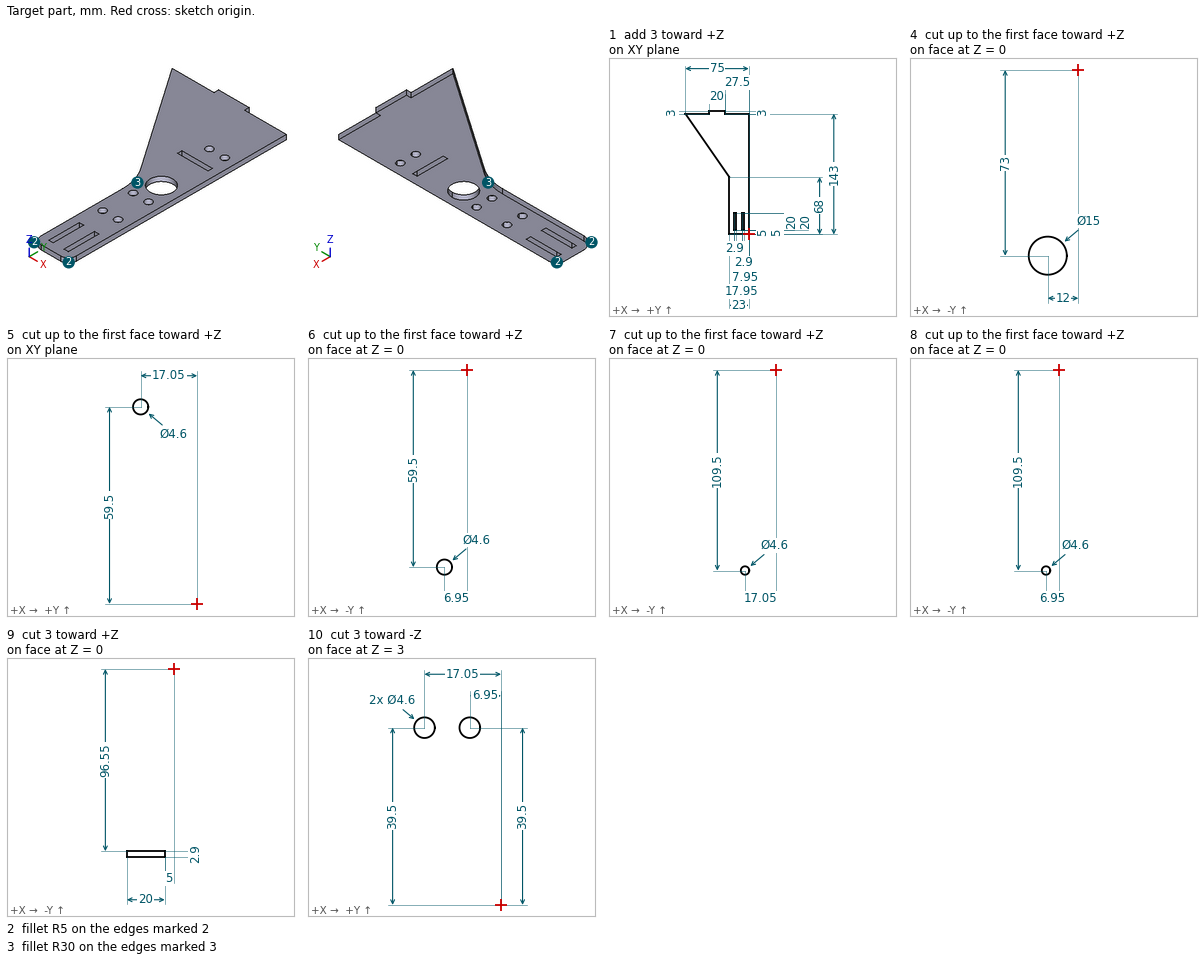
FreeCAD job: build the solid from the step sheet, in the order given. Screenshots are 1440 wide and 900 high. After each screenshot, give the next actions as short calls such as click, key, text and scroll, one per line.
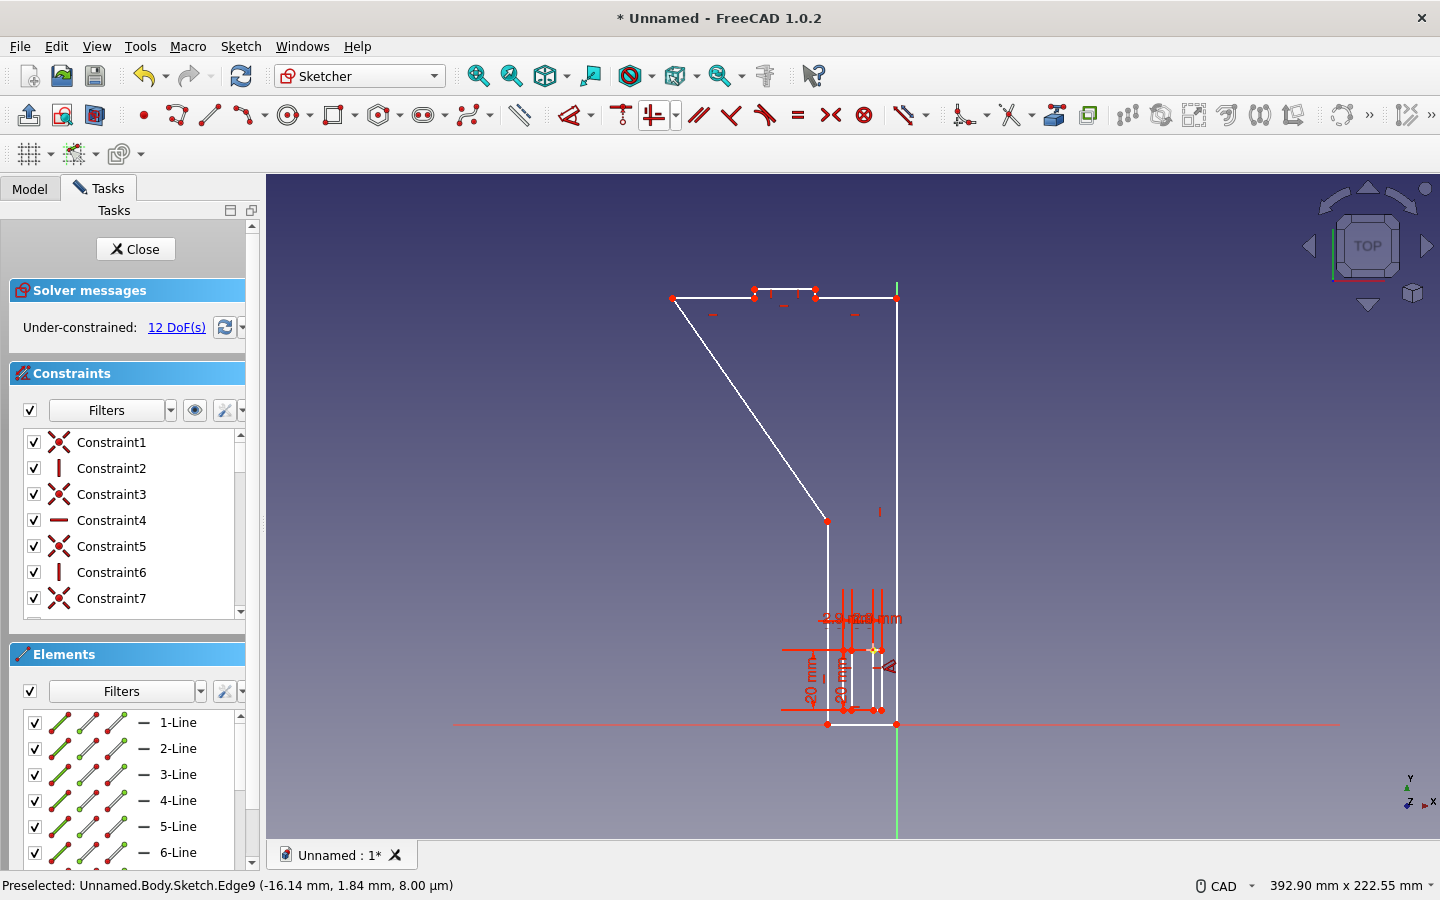
scroll(815, 294, up, 8)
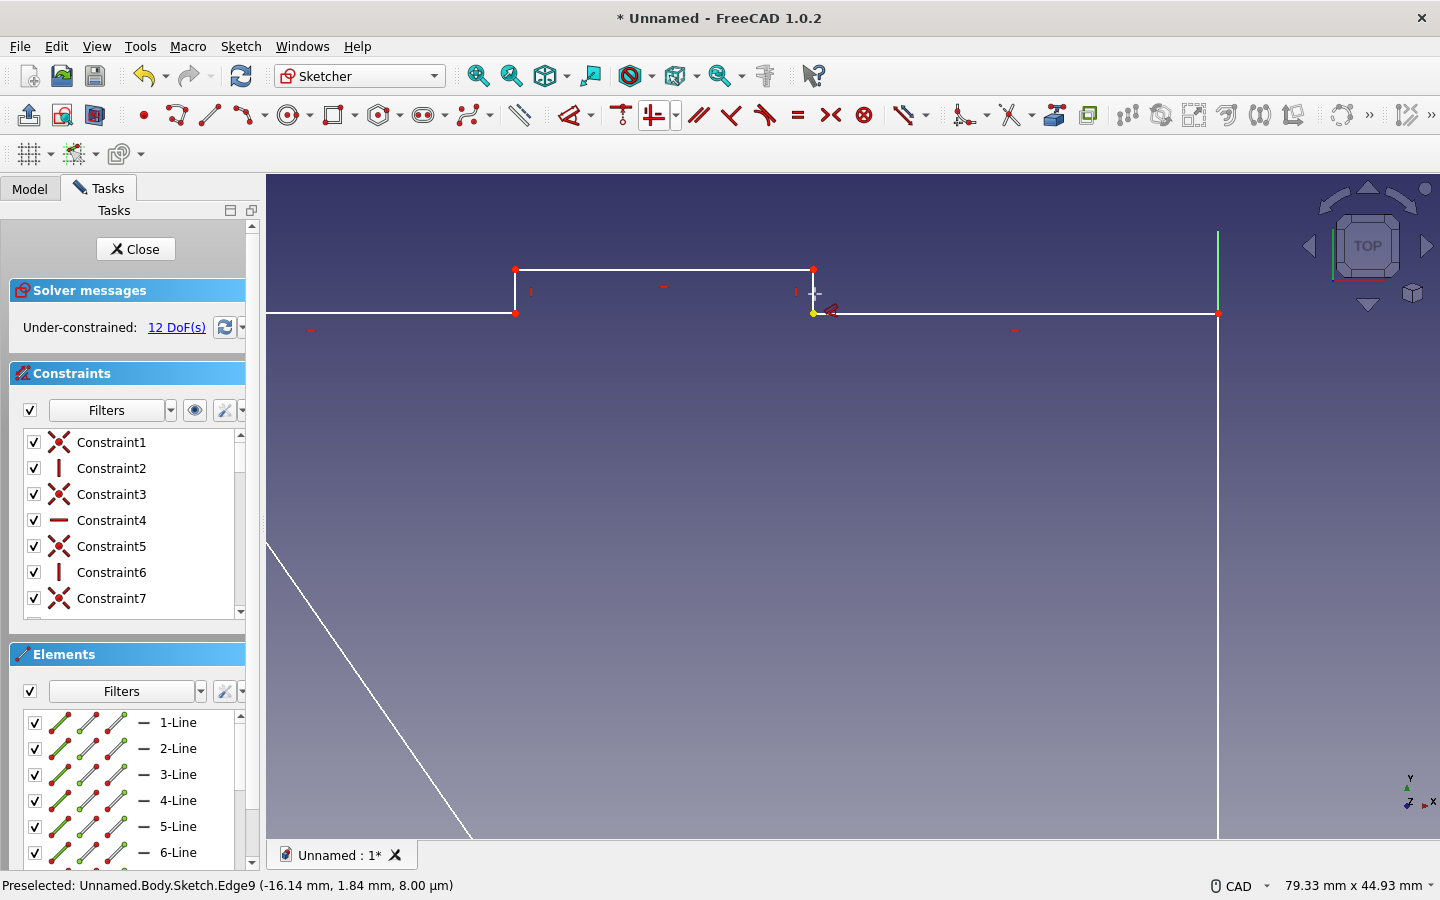
click(813, 292)
click(847, 292)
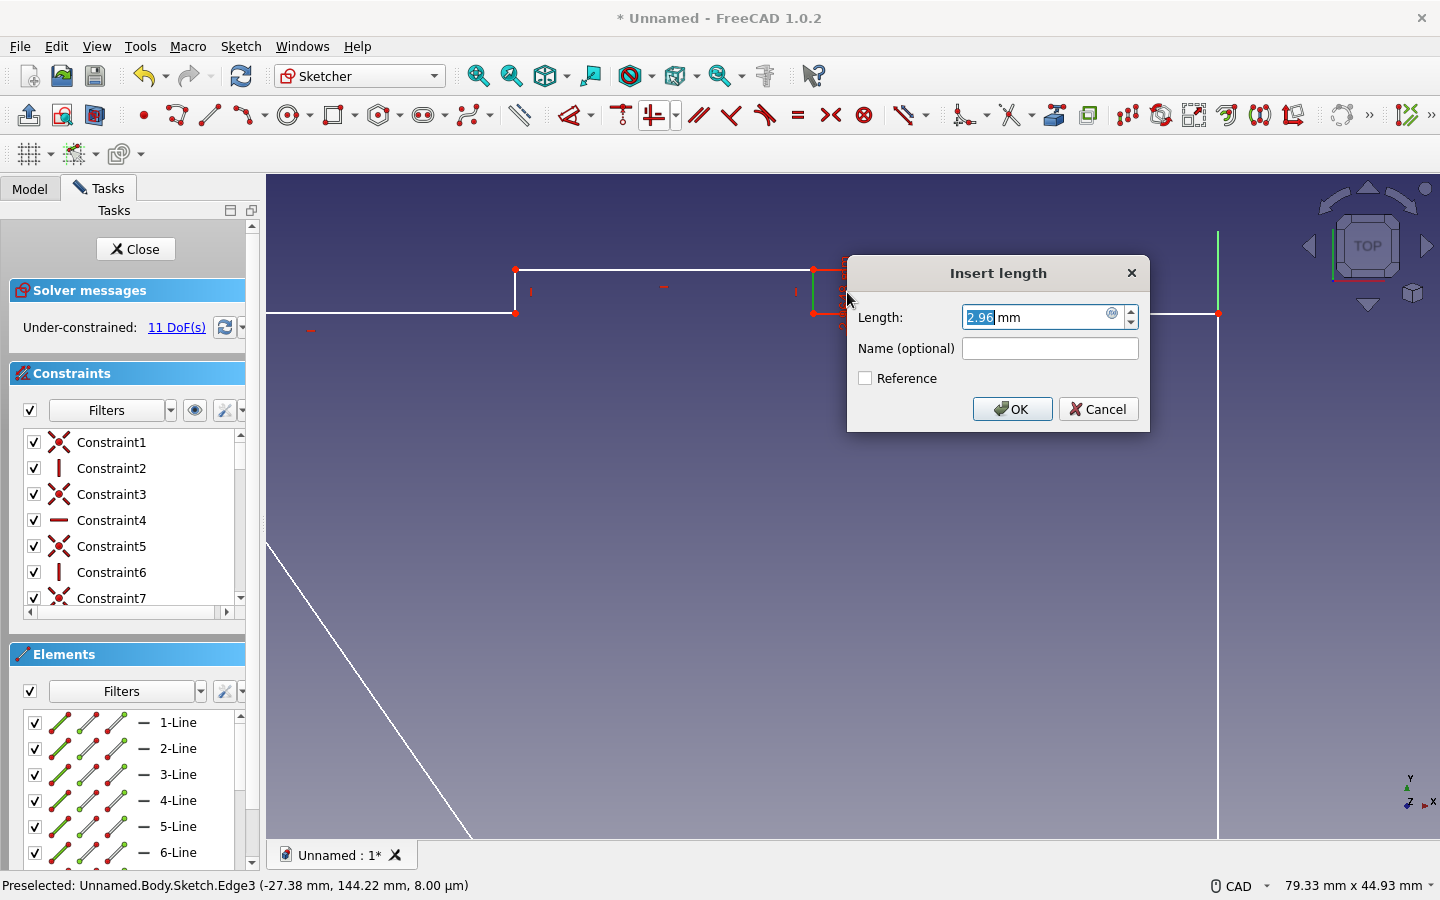
text(3)
key(Return)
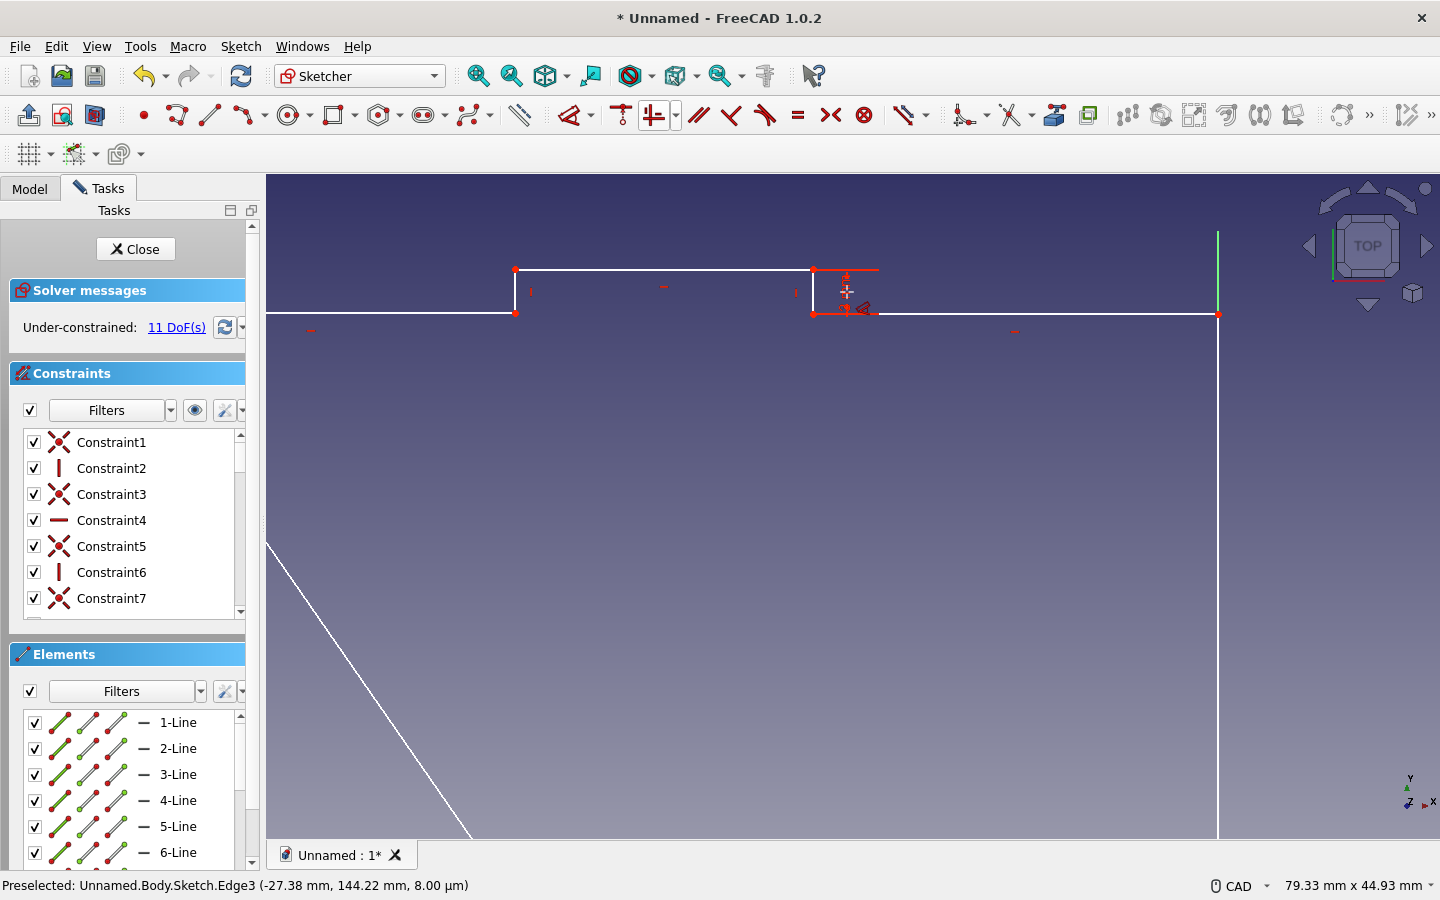
click(515, 283)
click(481, 292)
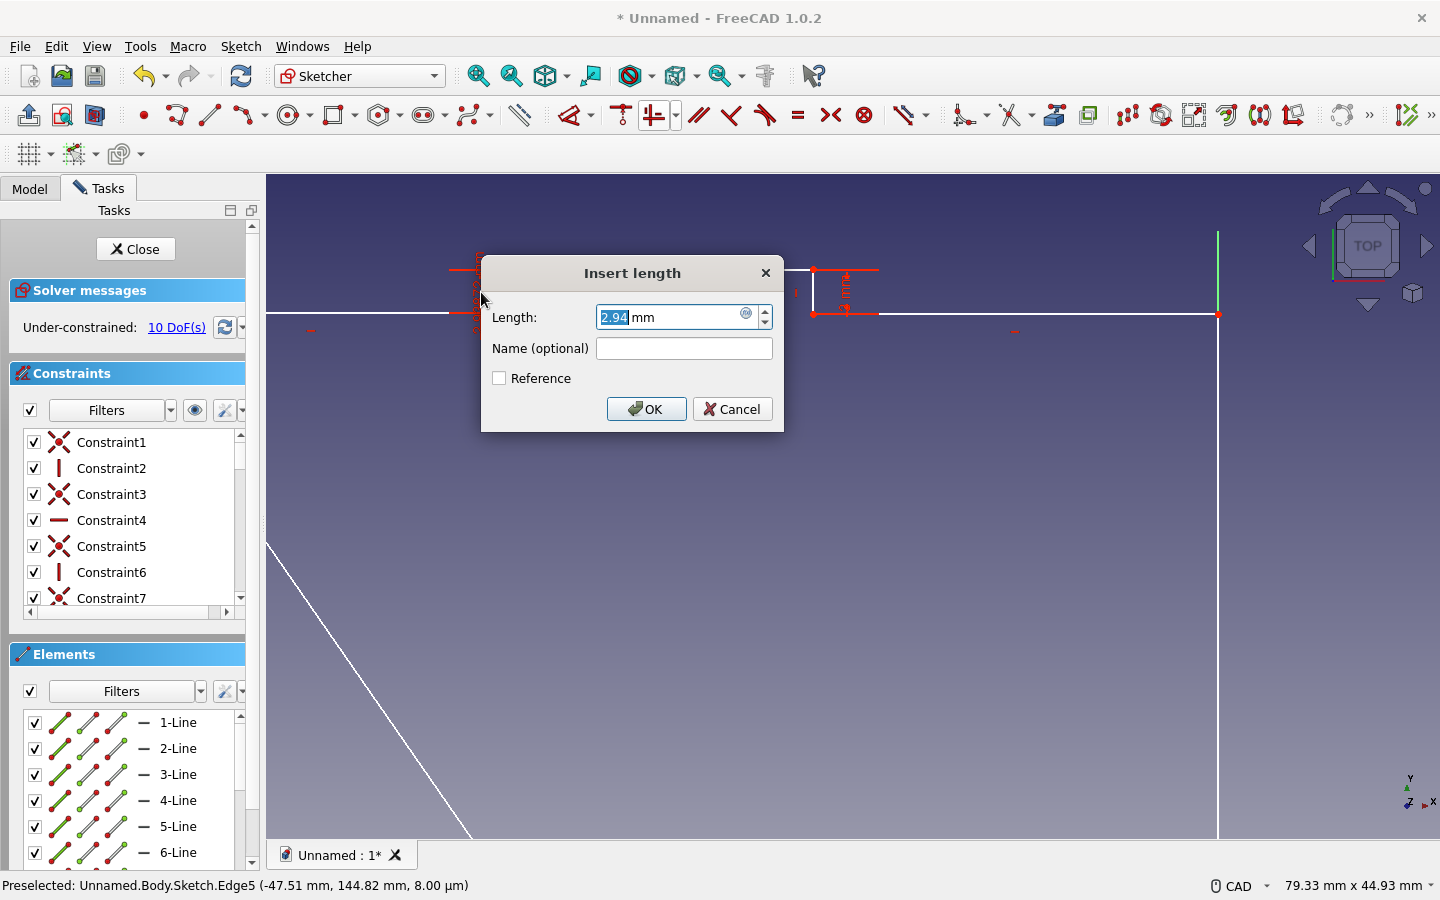
text(3)
key(Return)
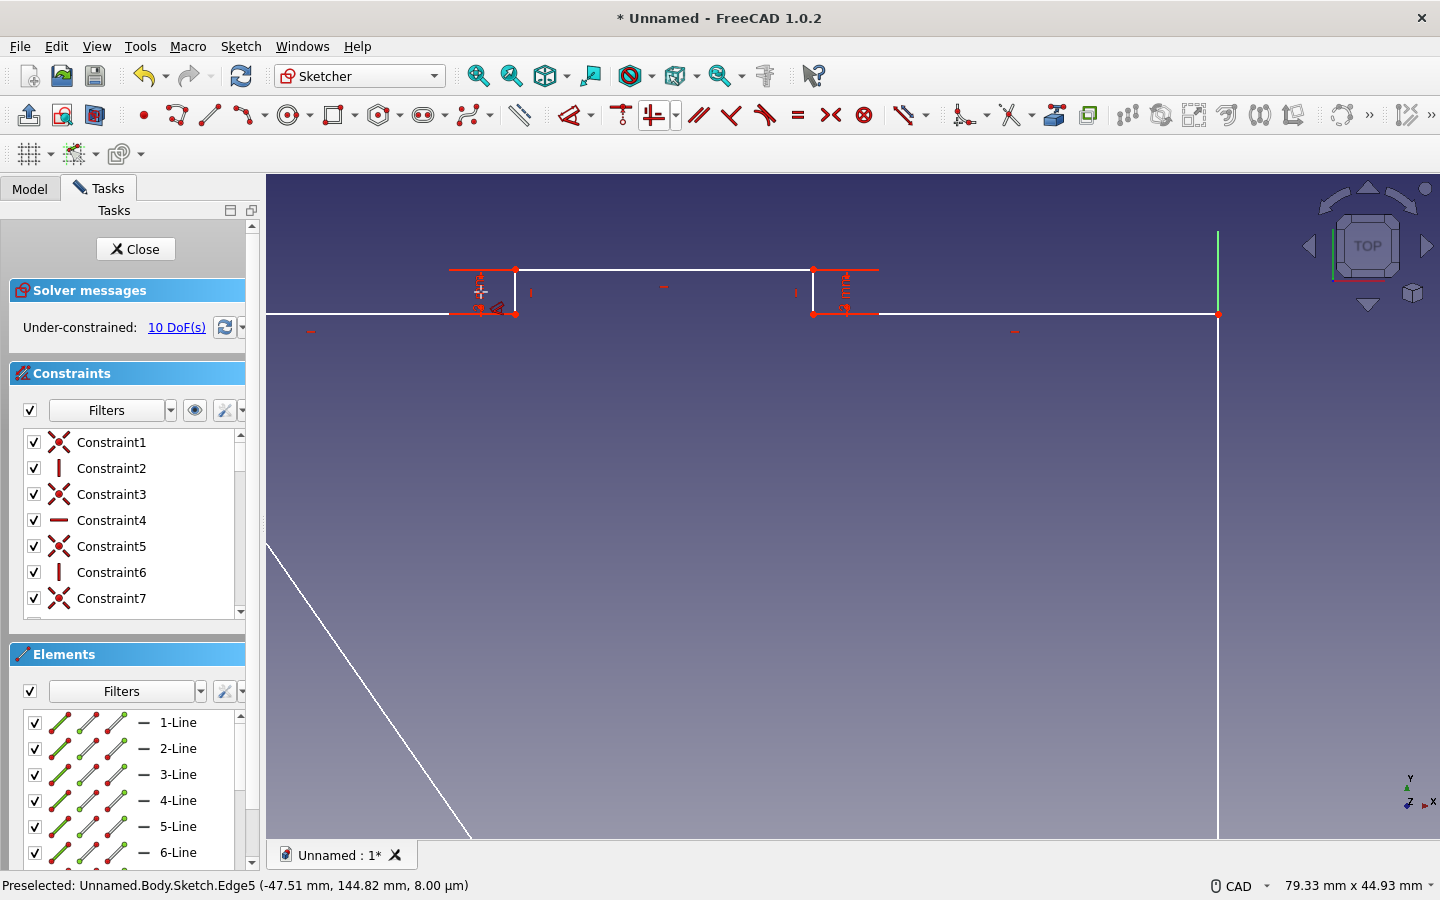
scroll(815, 294, down, 8)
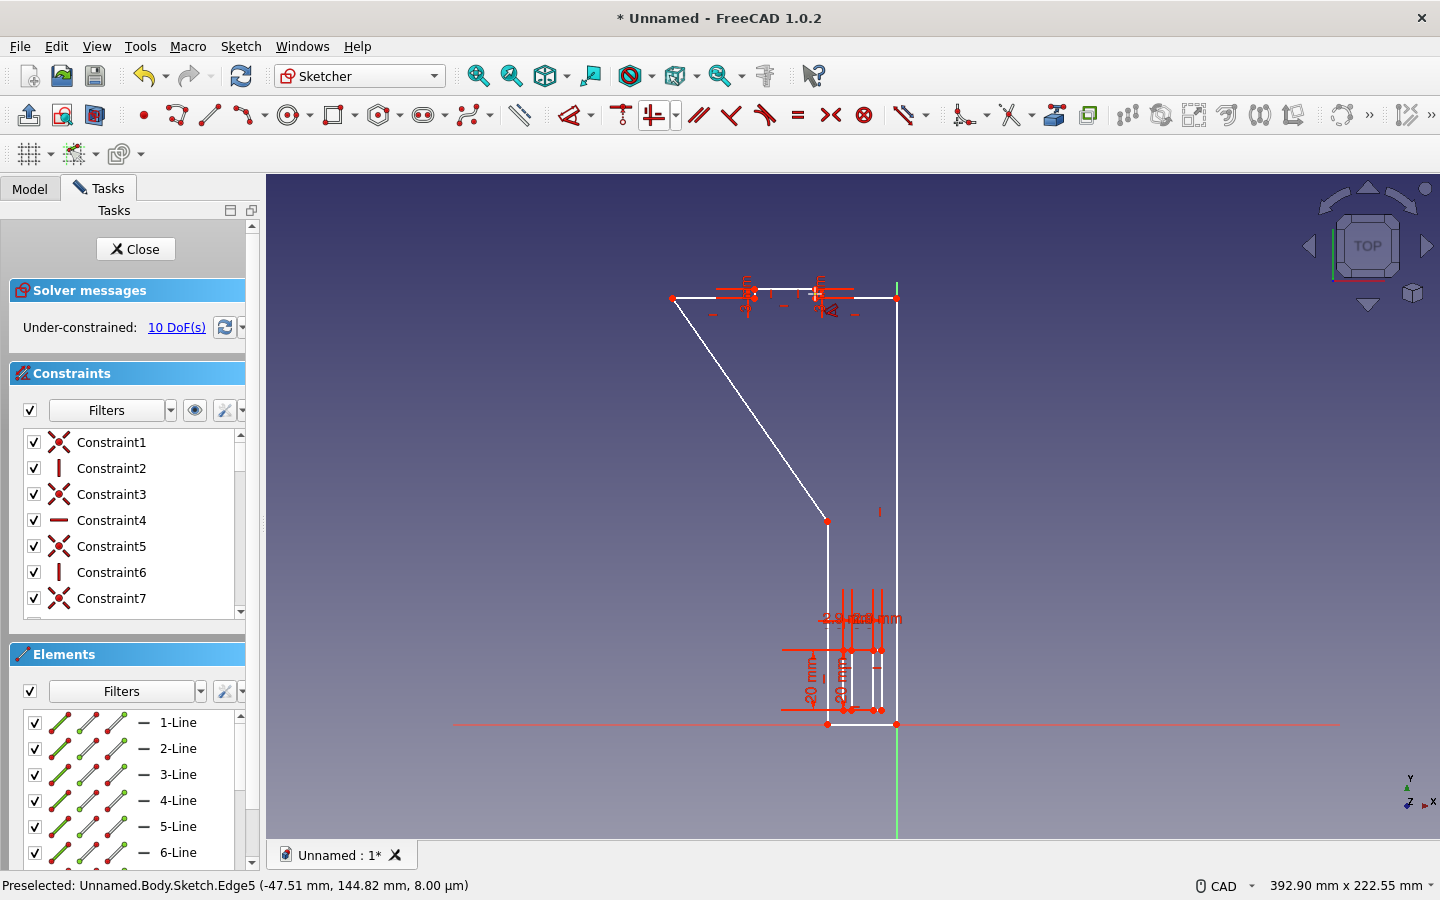
click(797, 289)
click(785, 255)